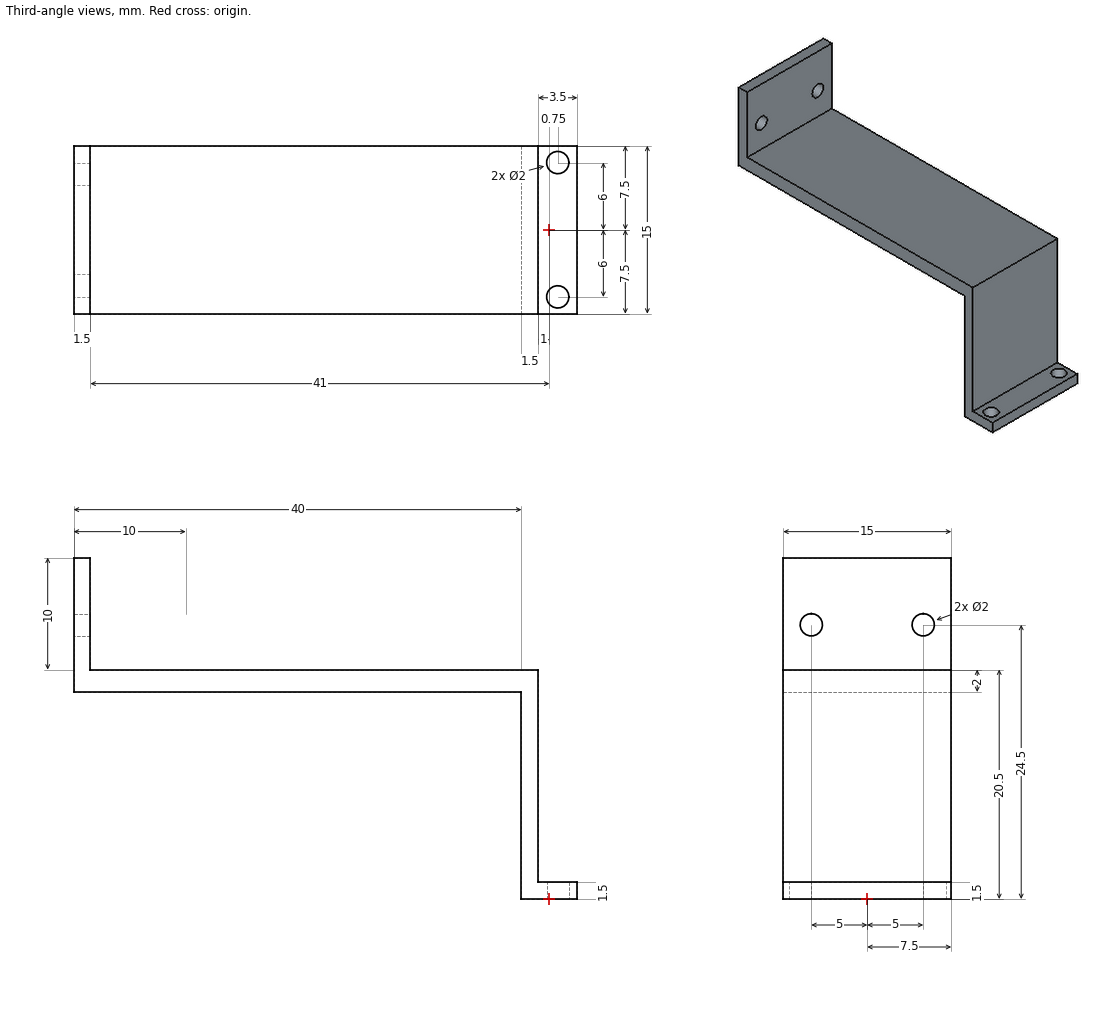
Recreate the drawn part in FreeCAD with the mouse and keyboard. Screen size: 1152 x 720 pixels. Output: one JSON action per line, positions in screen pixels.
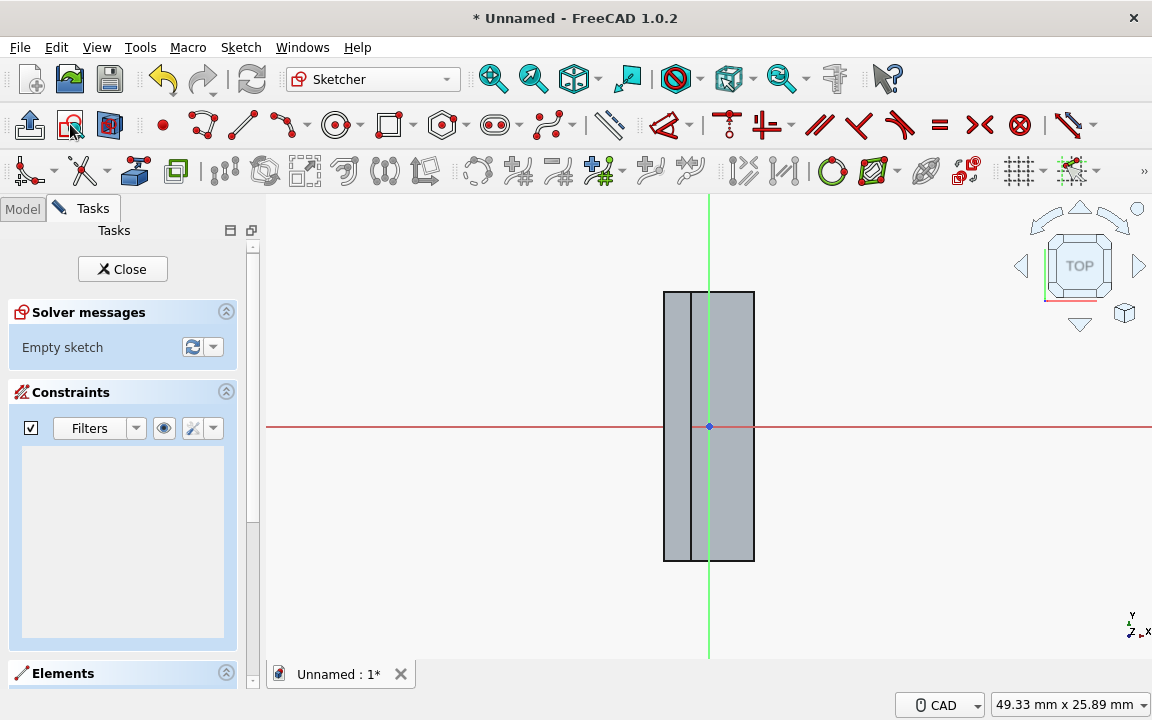
{"action": "left_click", "coordinate": [110, 126]}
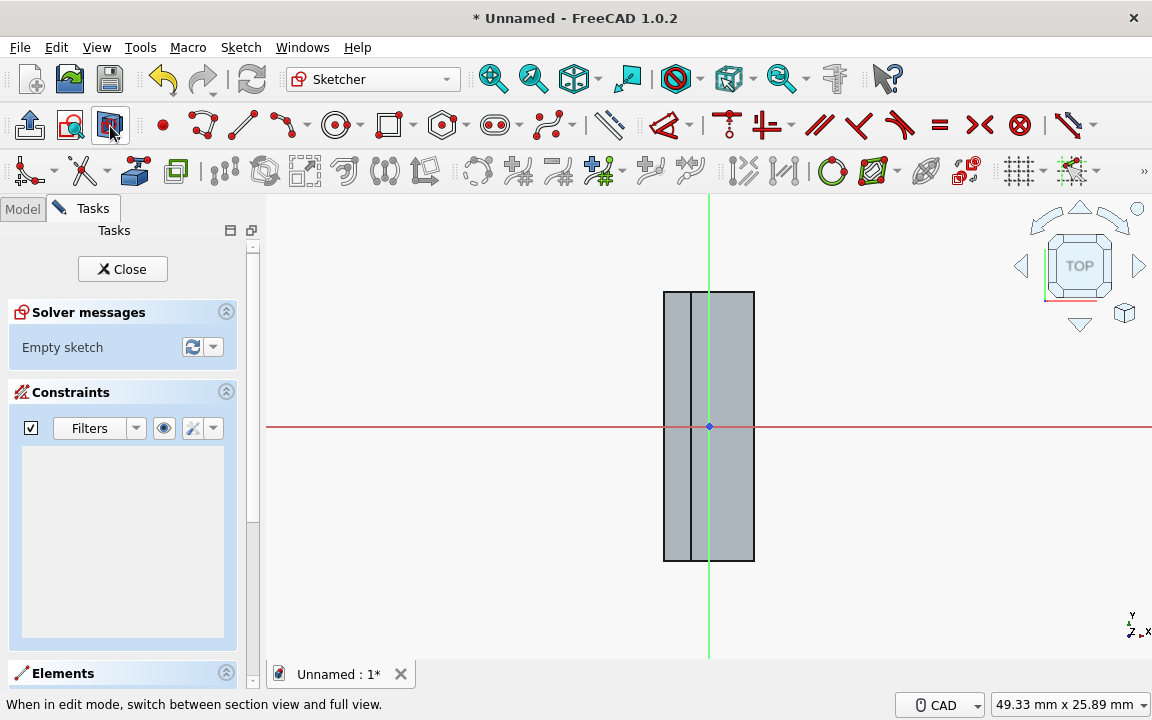
{"action": "left_click", "coordinate": [336, 126]}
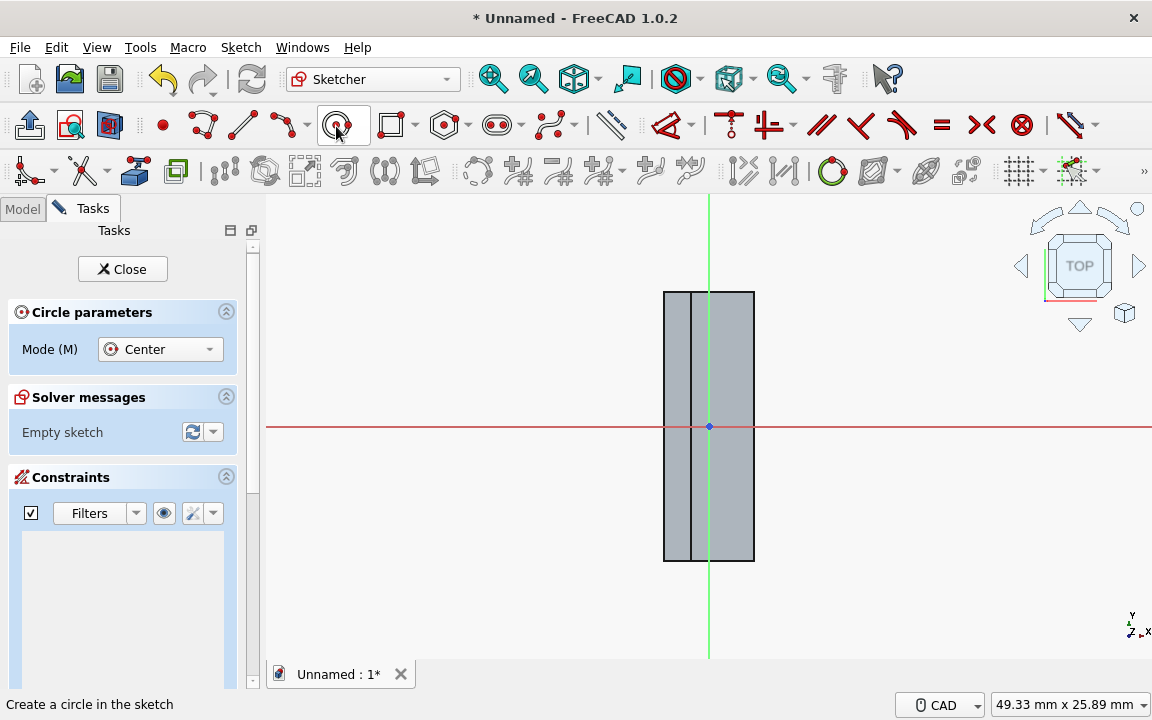
{"action": "scroll", "coordinate": [722, 319], "scroll_direction": "up", "scroll_amount": 2}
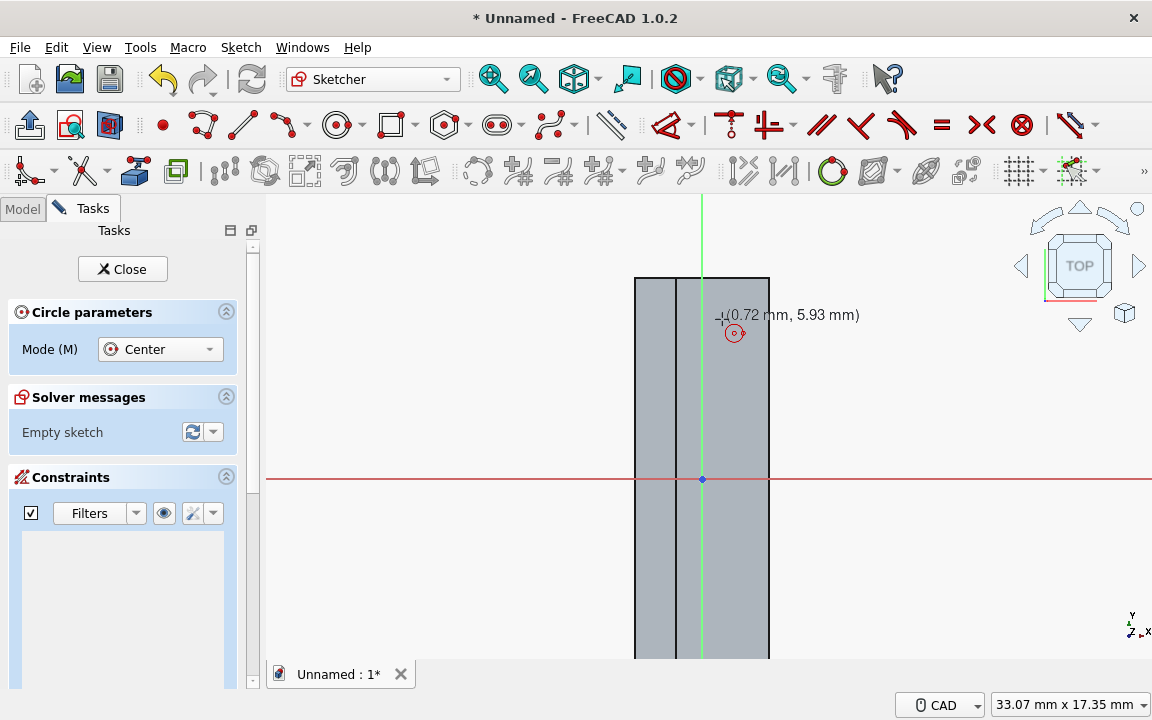
{"action": "left_click", "coordinate": [722, 318]}
{"action": "left_click", "coordinate": [741, 300]}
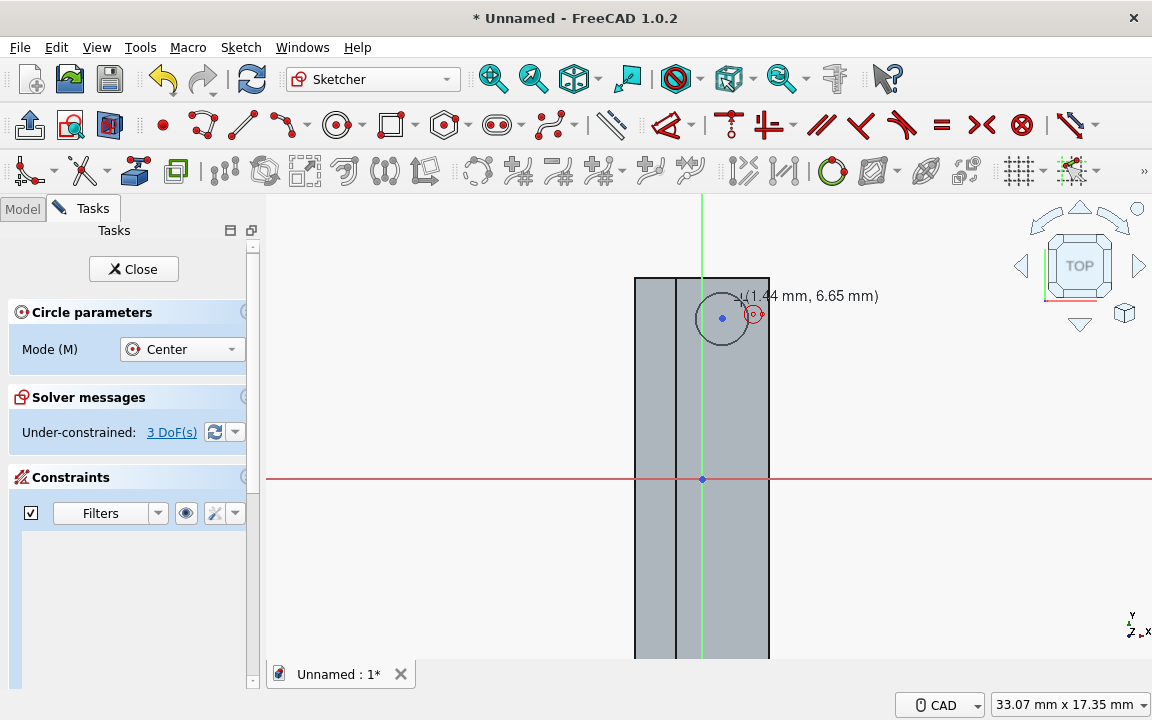
{"action": "scroll", "coordinate": [294, 222], "scroll_direction": "down", "scroll_amount": 1}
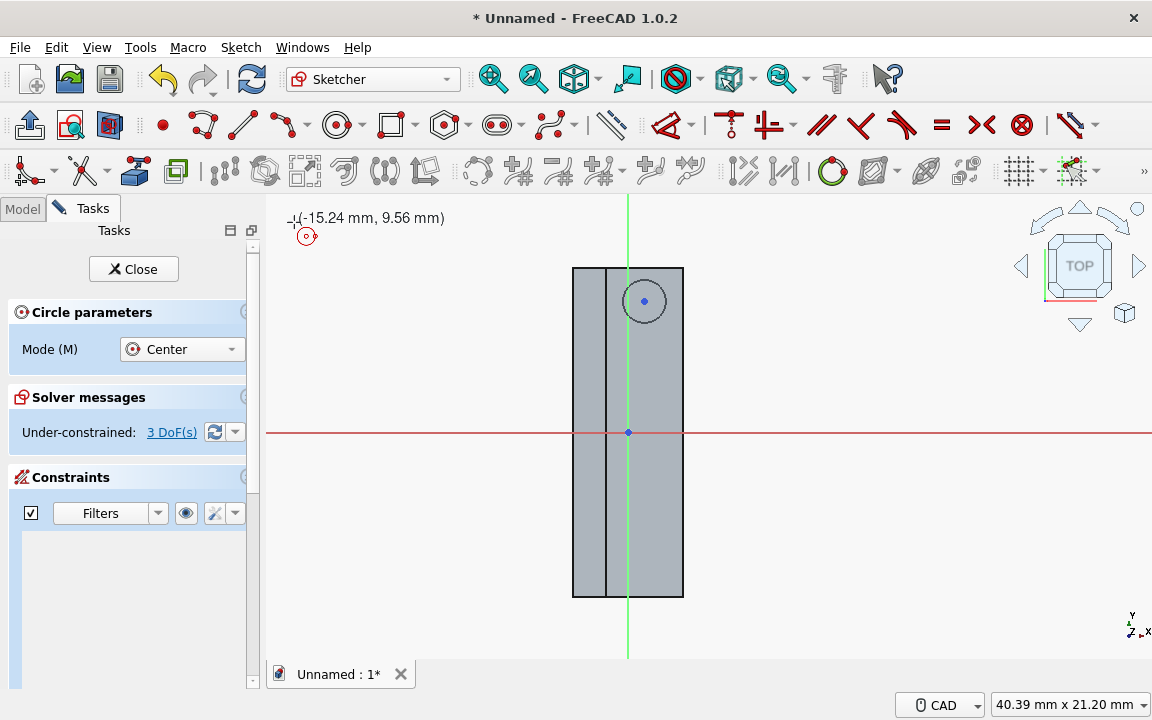
{"action": "left_click", "coordinate": [645, 564]}
{"action": "left_click", "coordinate": [660, 549]}
{"action": "key", "text": "Escape"}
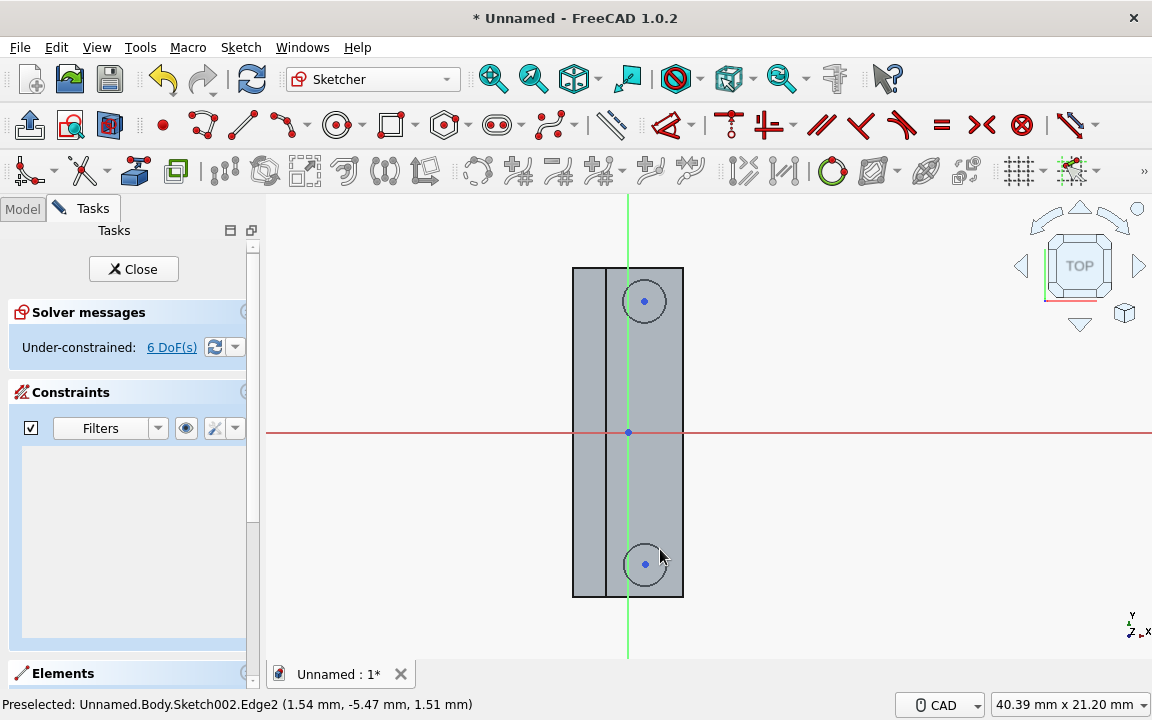
{"action": "left_click", "coordinate": [660, 286]}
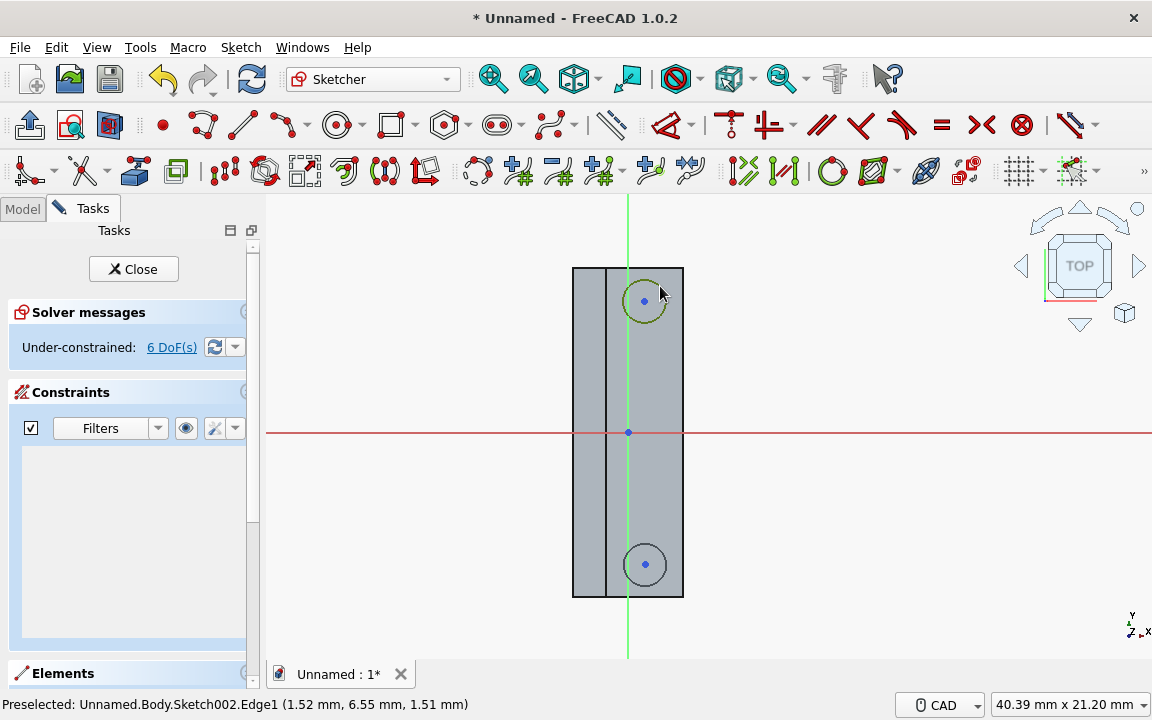
{"action": "left_click", "coordinate": [660, 550]}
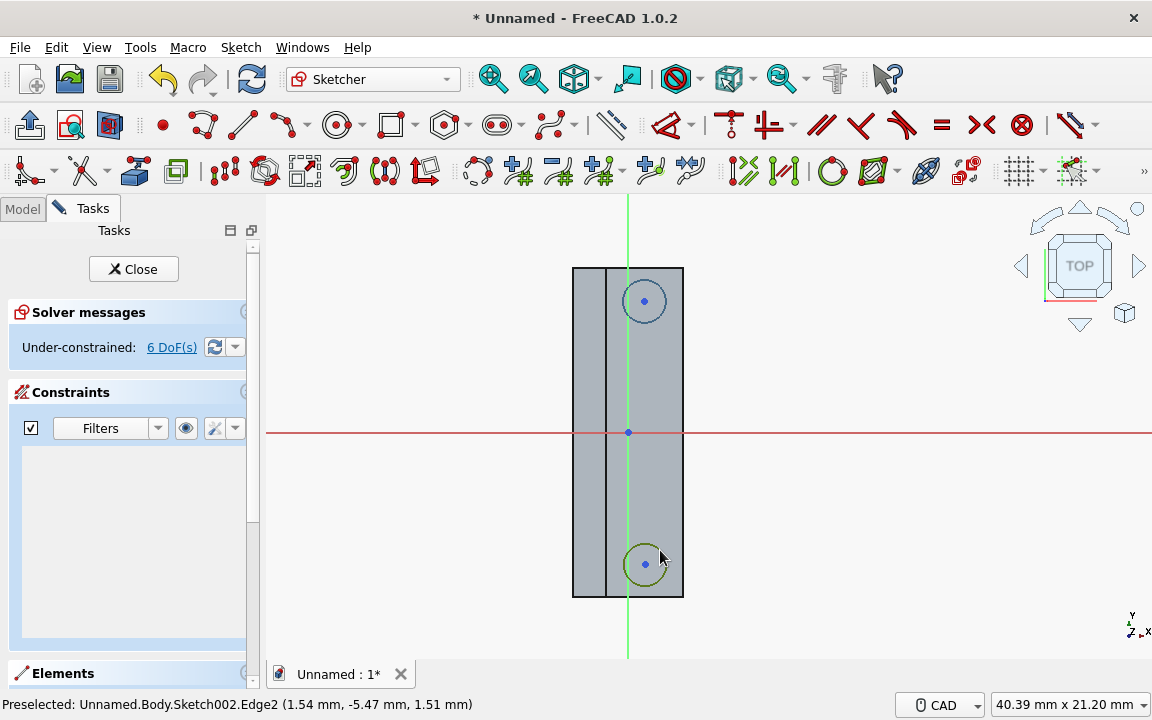
{"action": "left_click", "coordinate": [942, 126]}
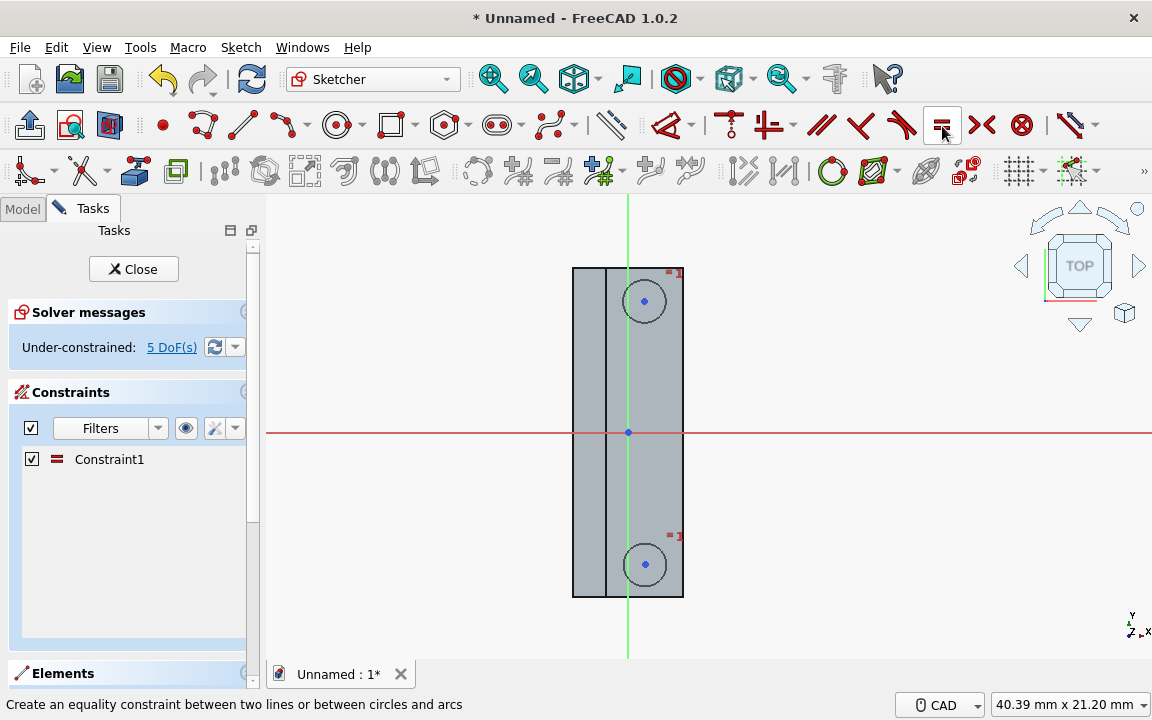
{"action": "left_click", "coordinate": [644, 301]}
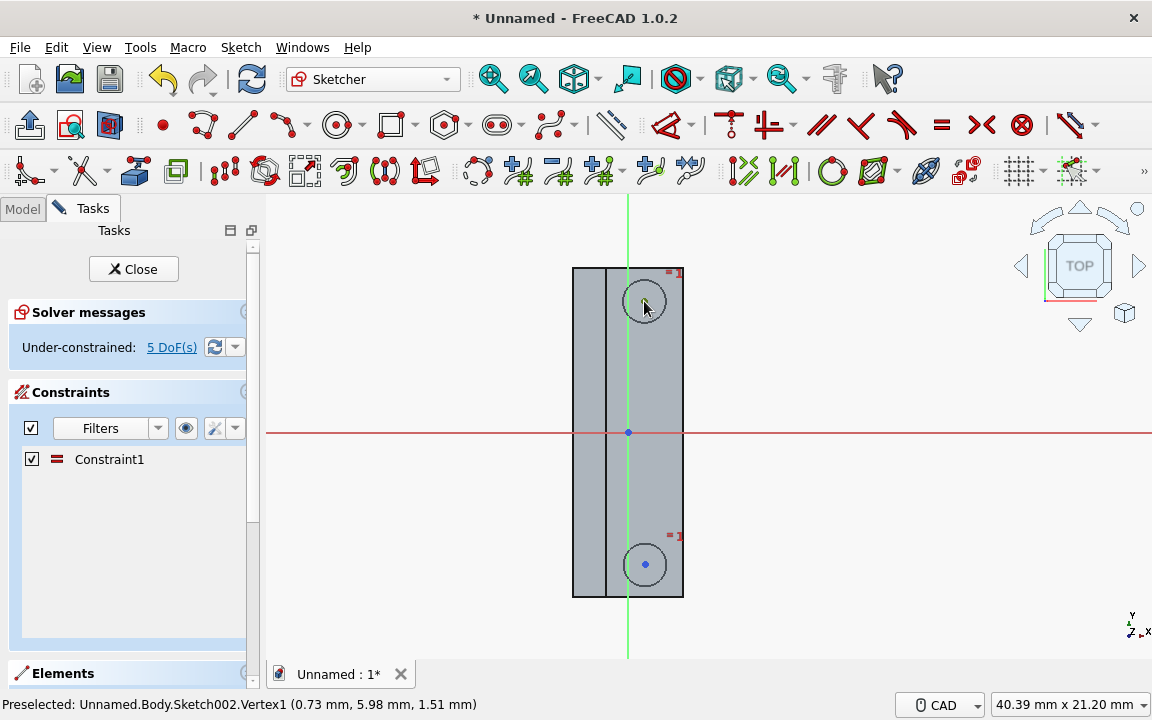
{"action": "left_click", "coordinate": [645, 565]}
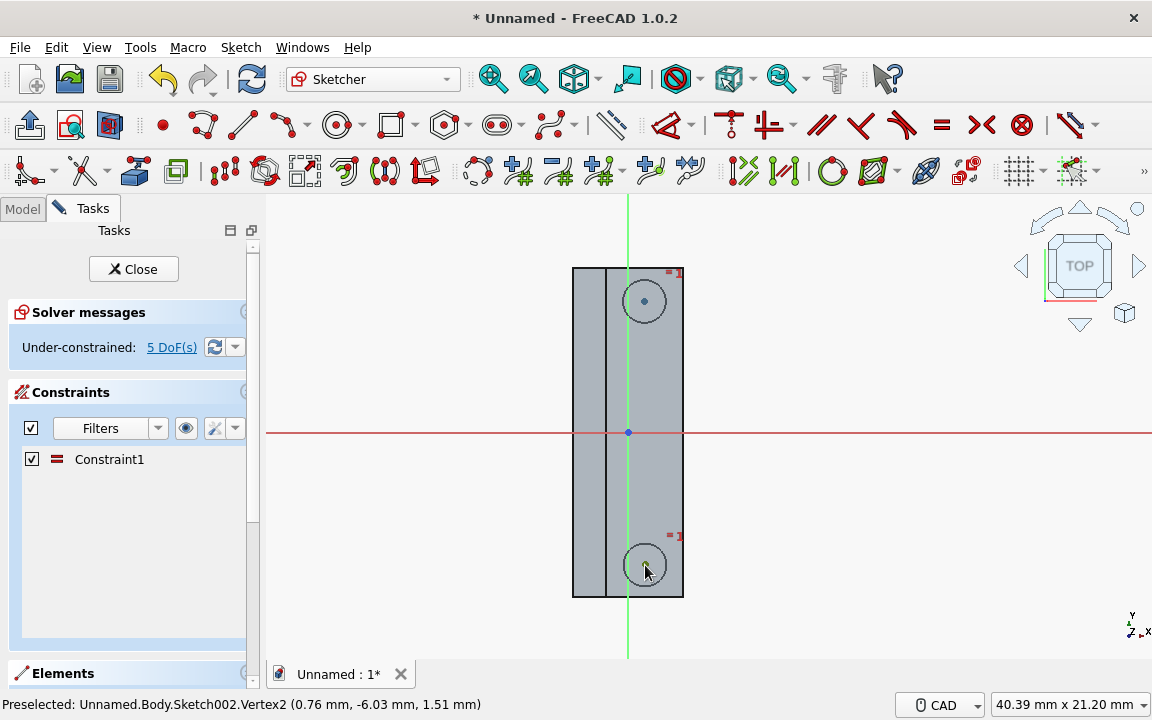
{"action": "left_click", "coordinate": [796, 126]}